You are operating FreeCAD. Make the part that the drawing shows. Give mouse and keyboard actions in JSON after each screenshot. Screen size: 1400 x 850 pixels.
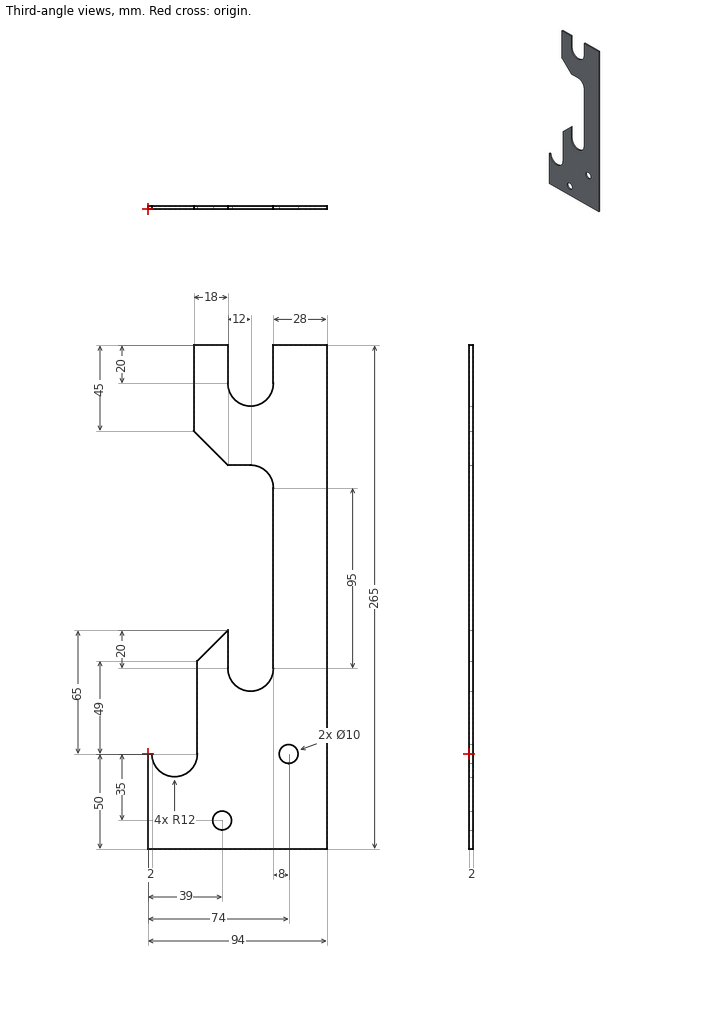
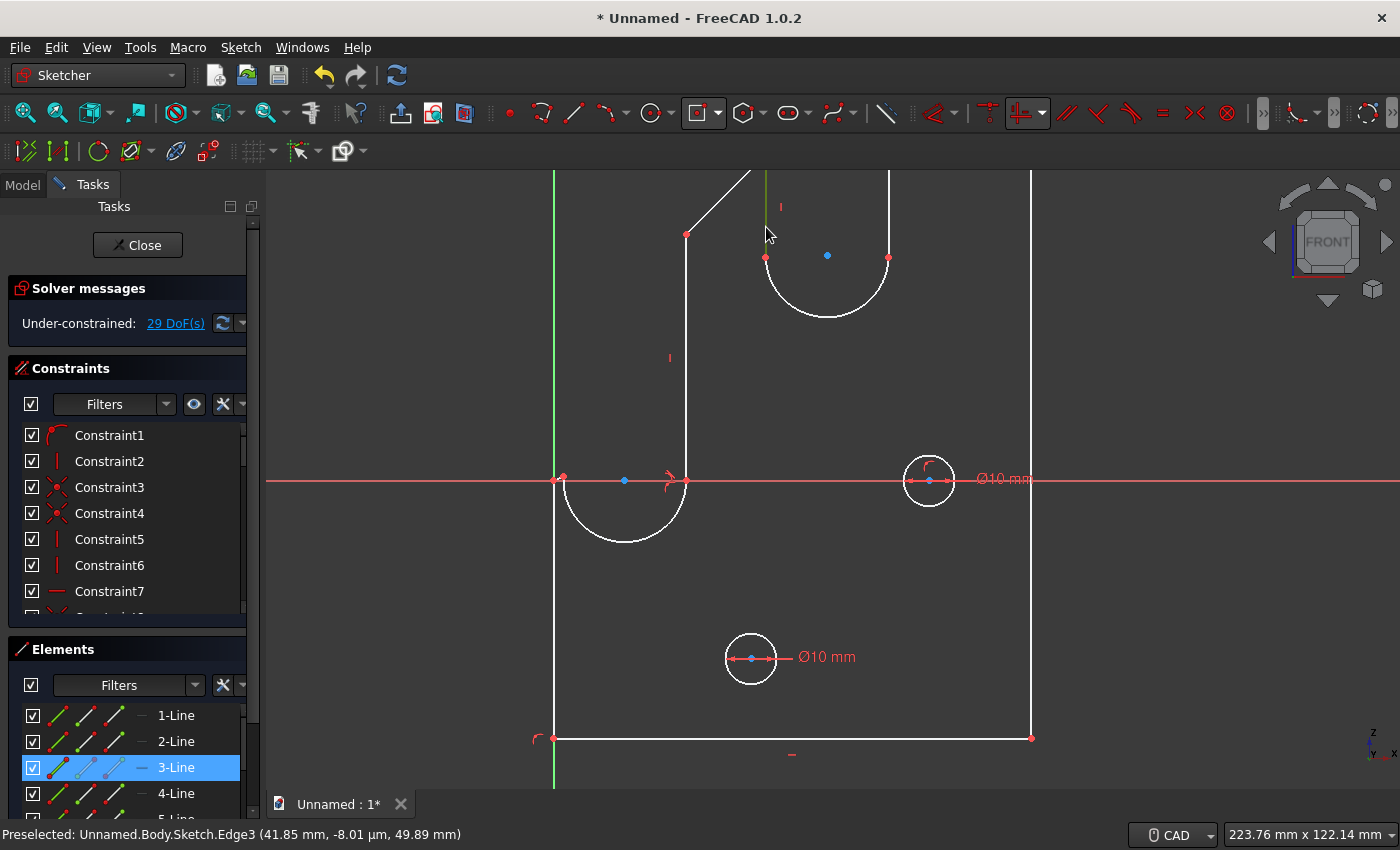
{"action": "left_click", "coordinate": [792, 306]}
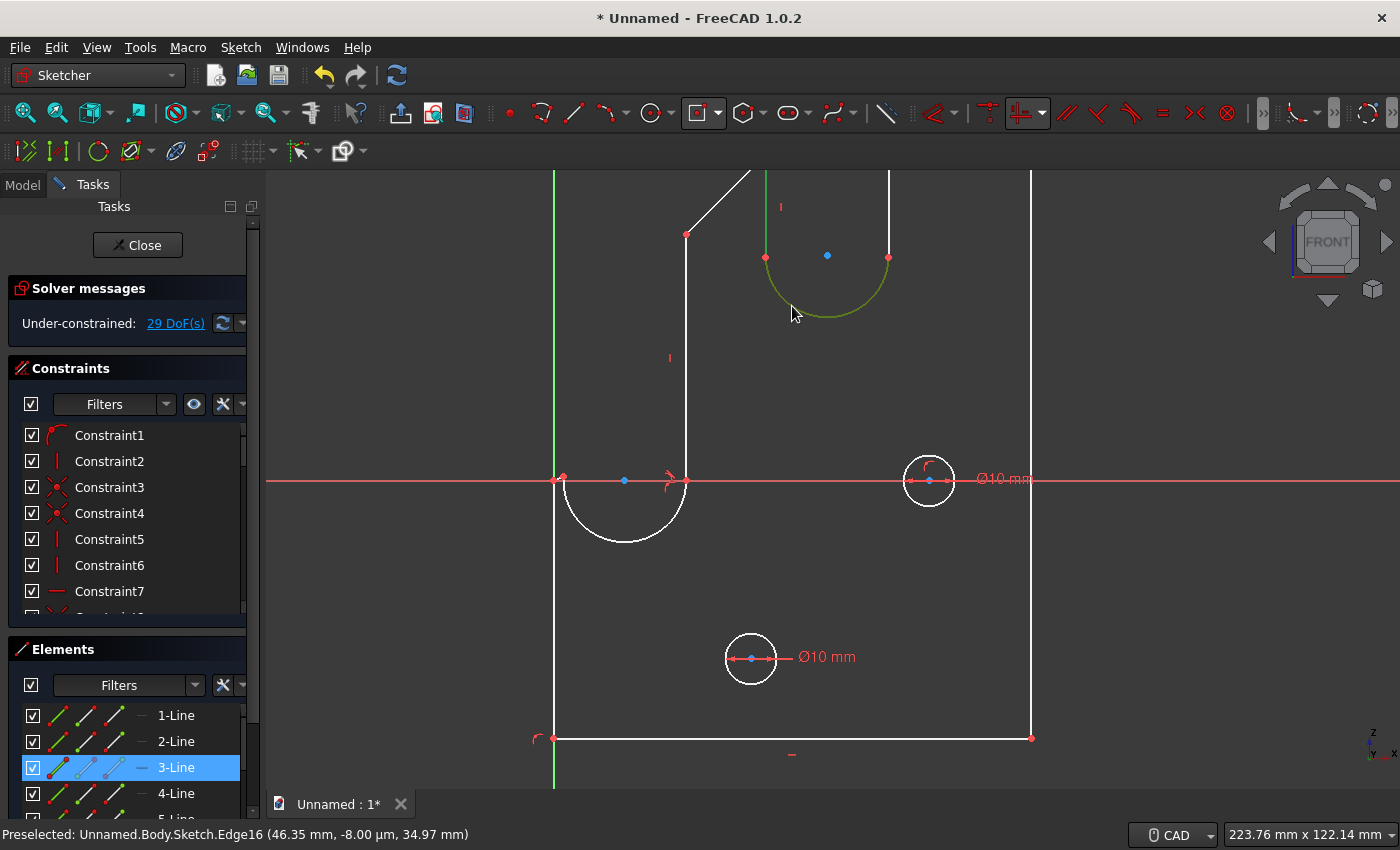
{"action": "key", "text": "t"}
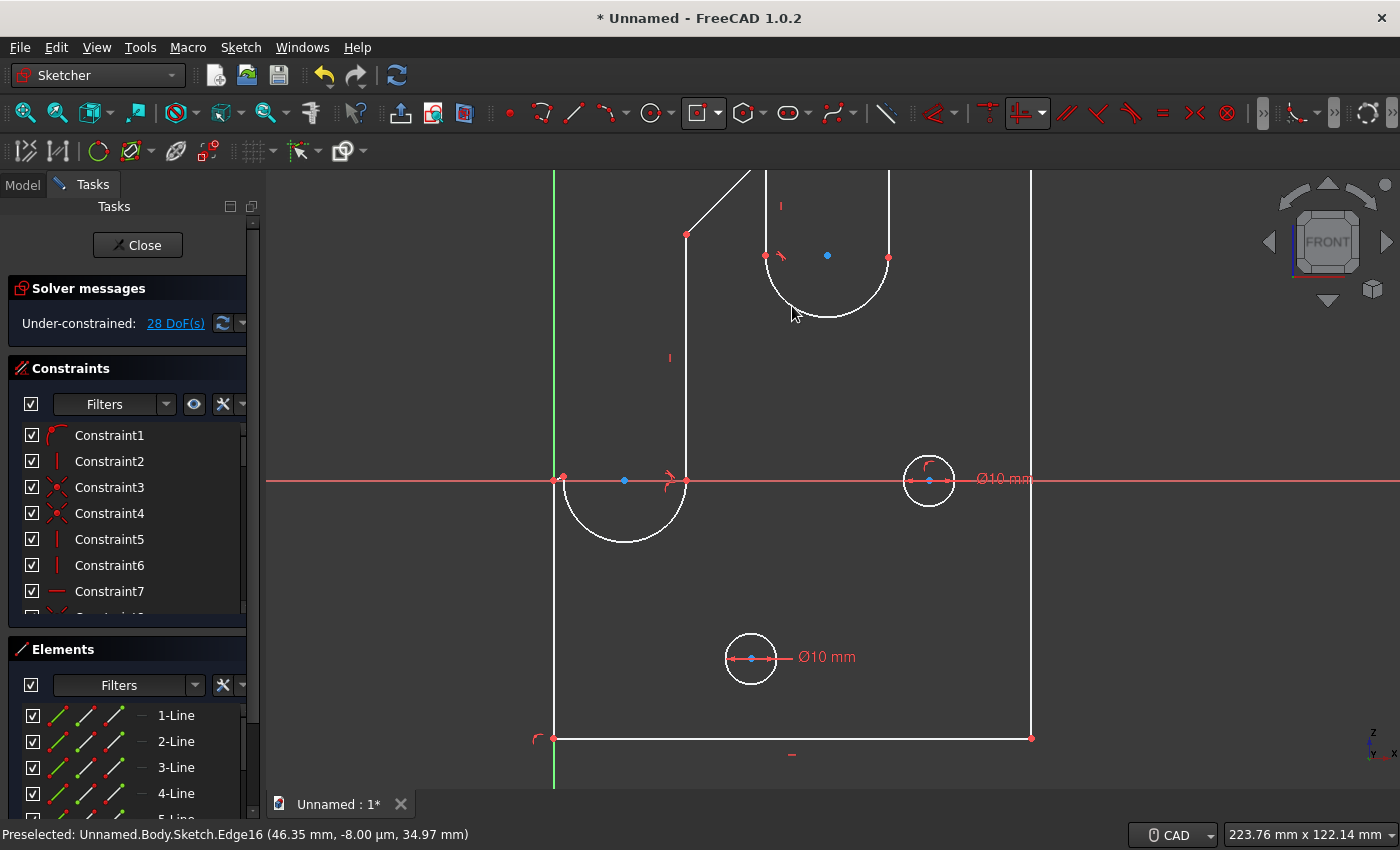
{"action": "scroll", "coordinate": [753, 659], "scroll_direction": "down", "scroll_amount": 6}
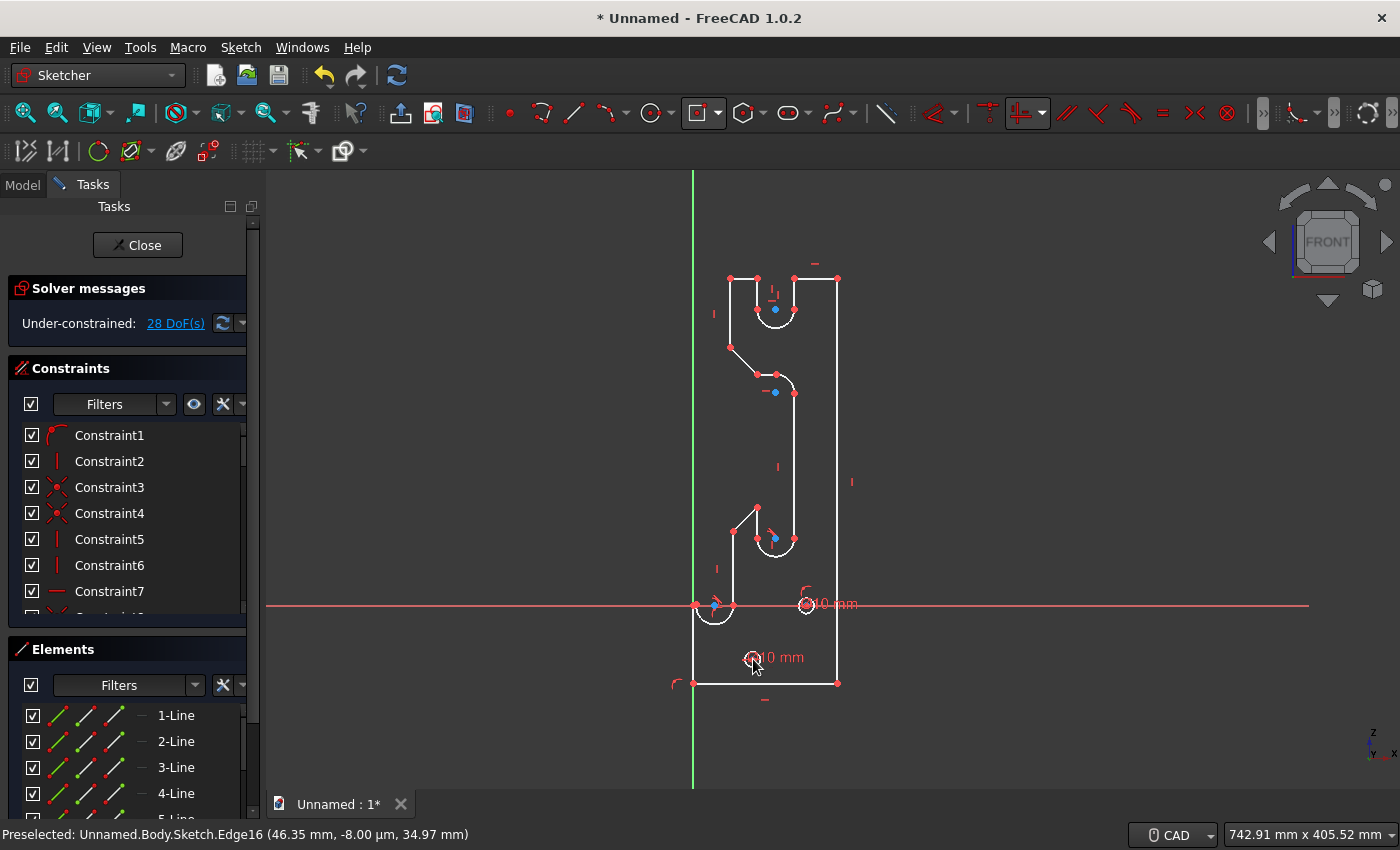
{"action": "left_click", "coordinate": [794, 495]}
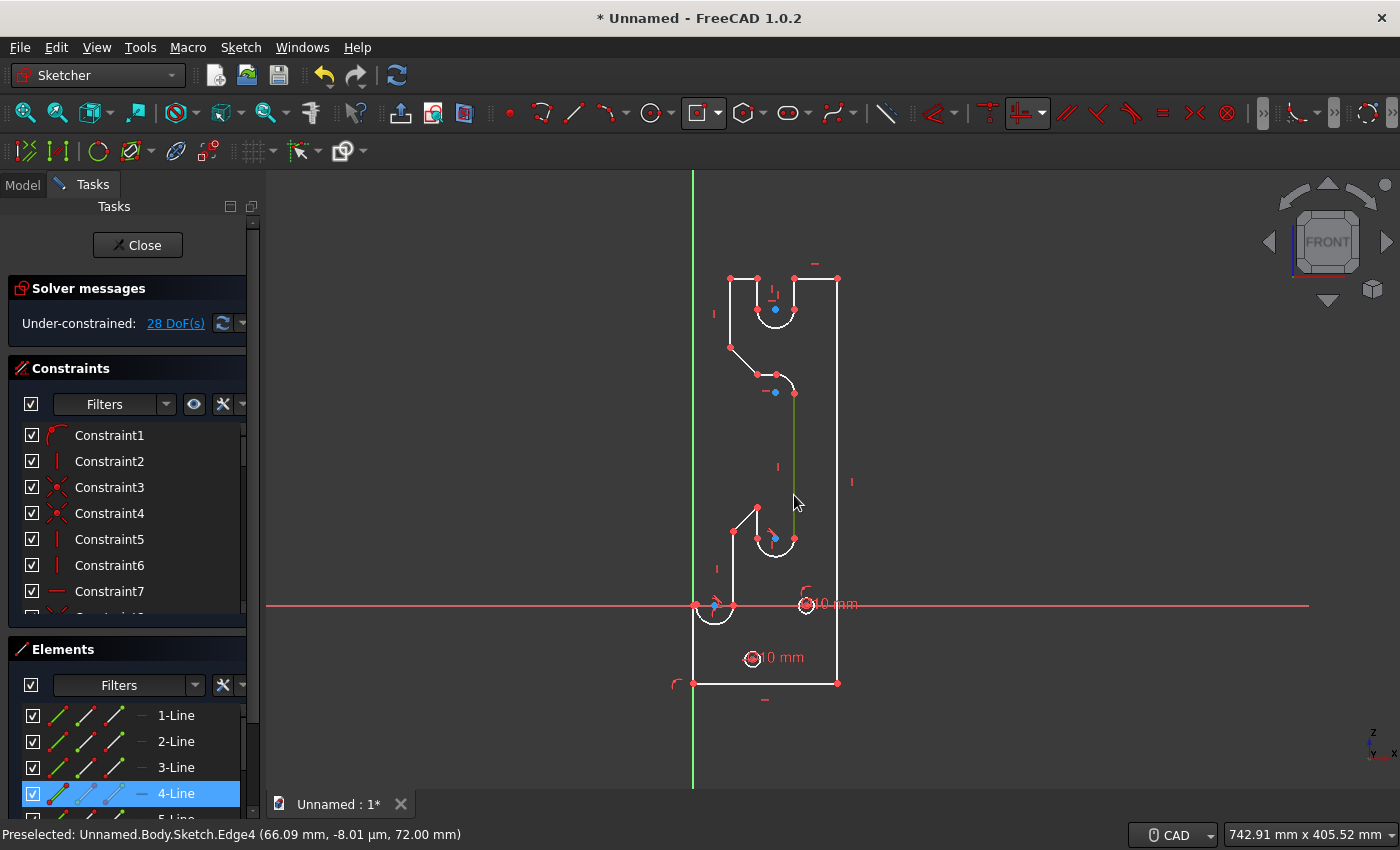
{"action": "left_click", "coordinate": [765, 553]}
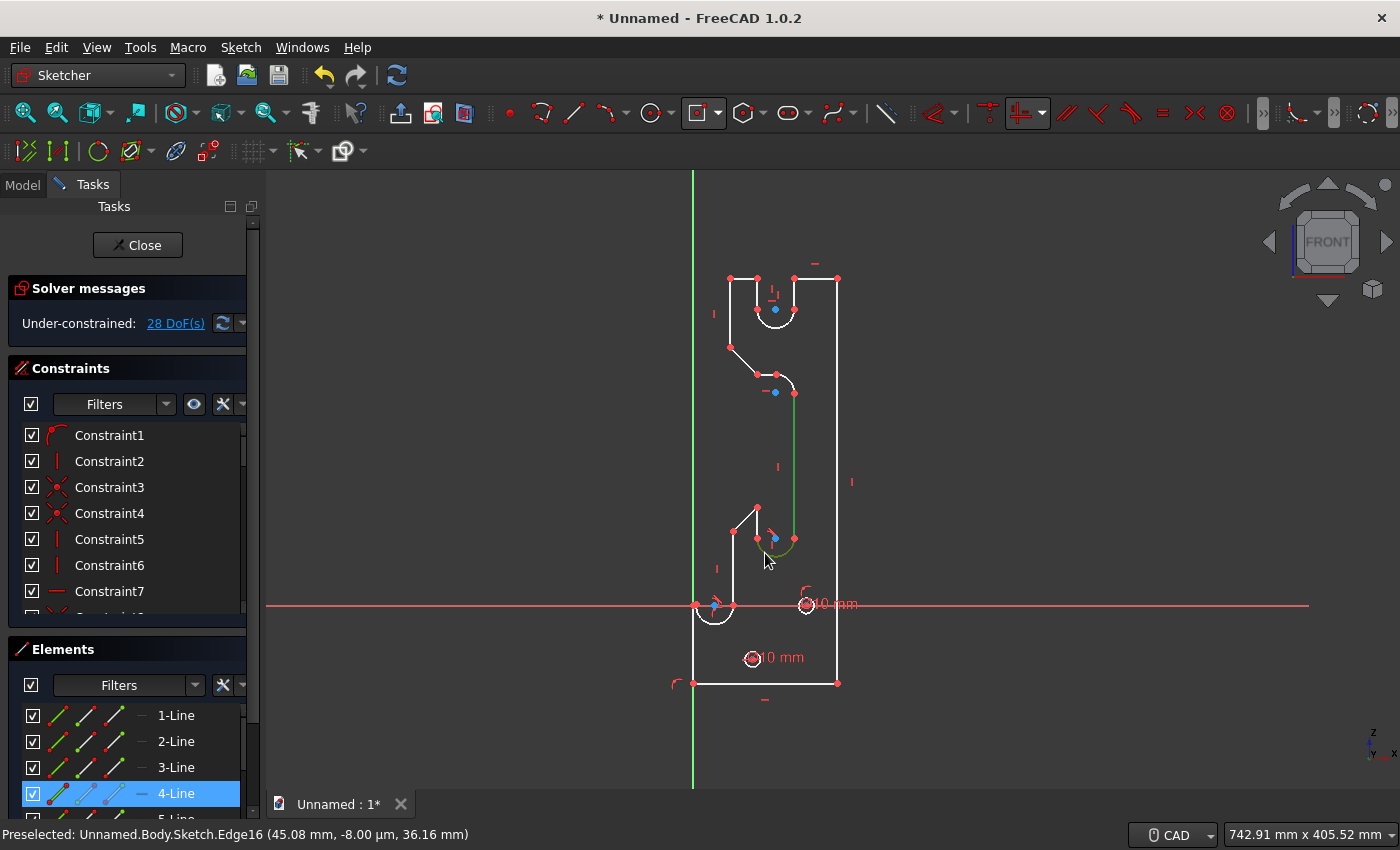
{"action": "key", "text": "t"}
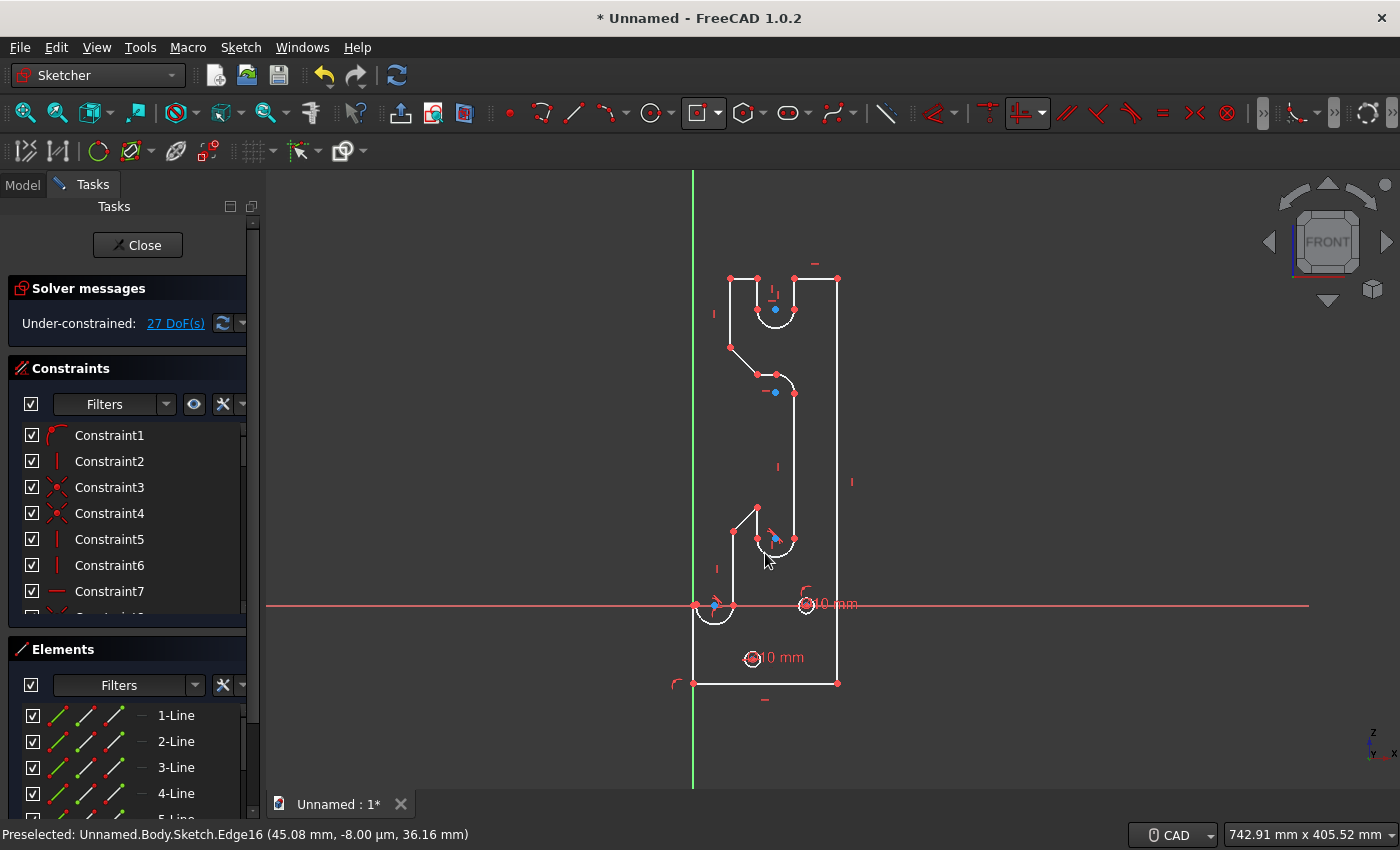
{"action": "left_click", "coordinate": [794, 495]}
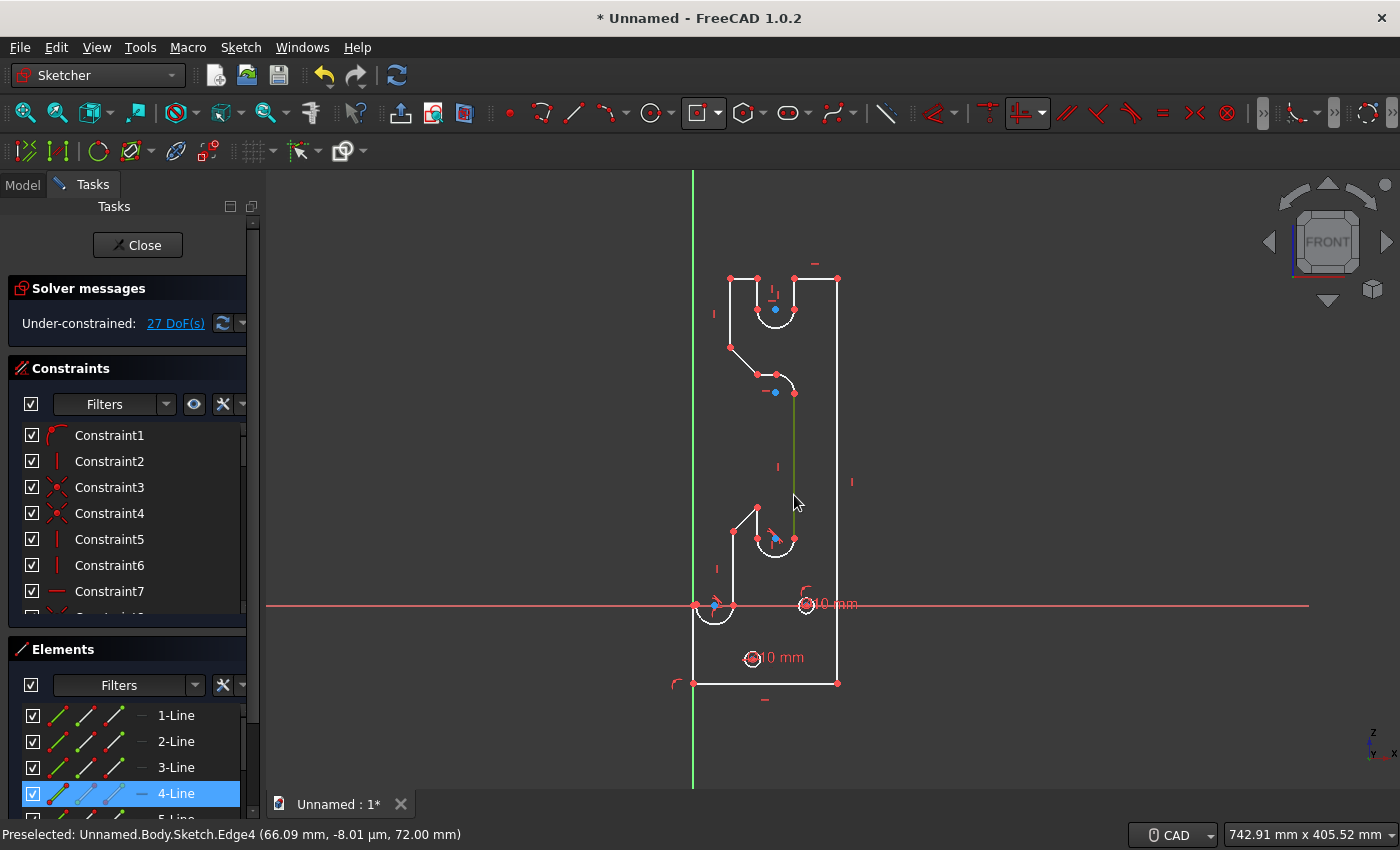
{"action": "left_click", "coordinate": [789, 380]}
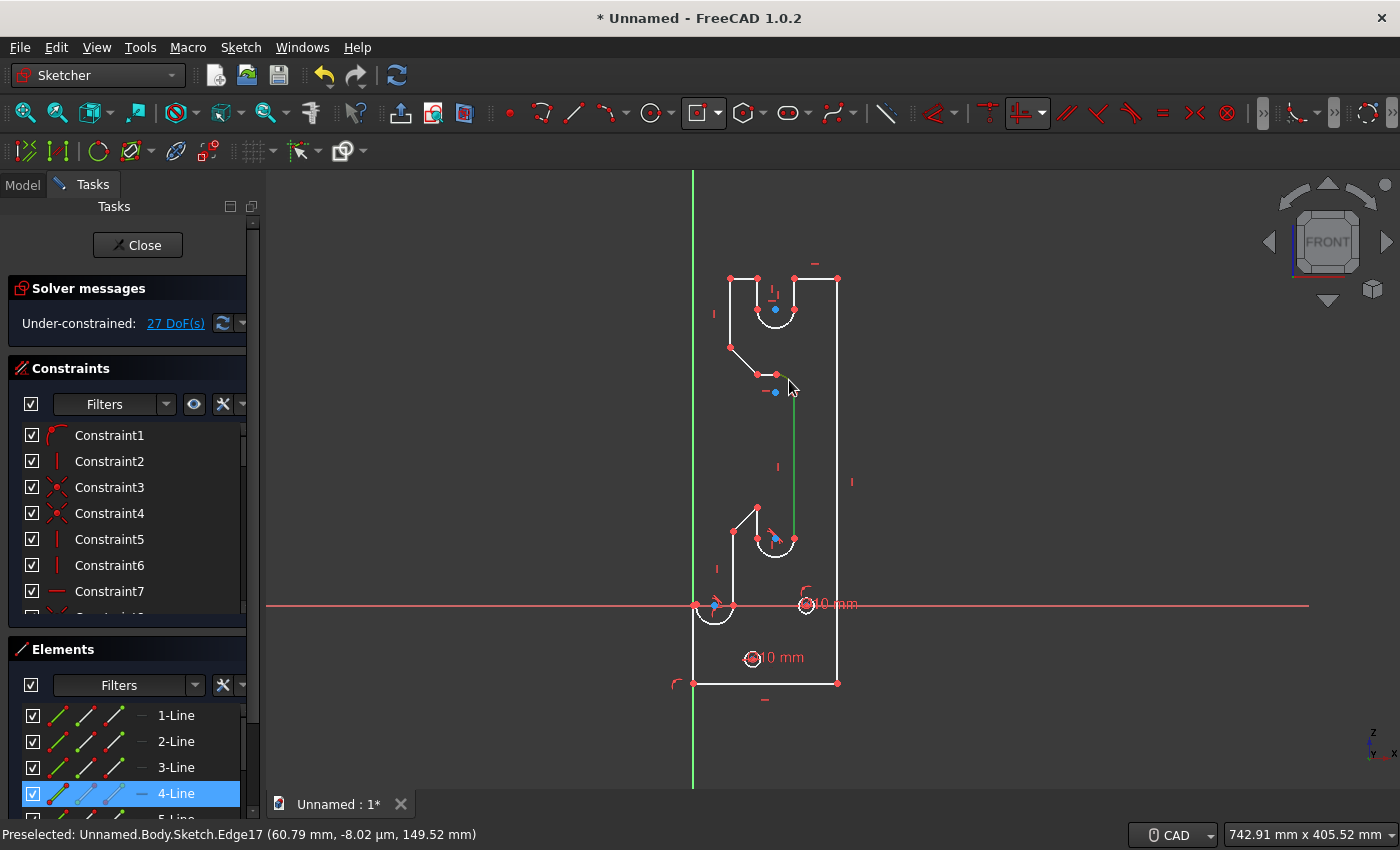
{"action": "left_click", "coordinate": [1132, 114]}